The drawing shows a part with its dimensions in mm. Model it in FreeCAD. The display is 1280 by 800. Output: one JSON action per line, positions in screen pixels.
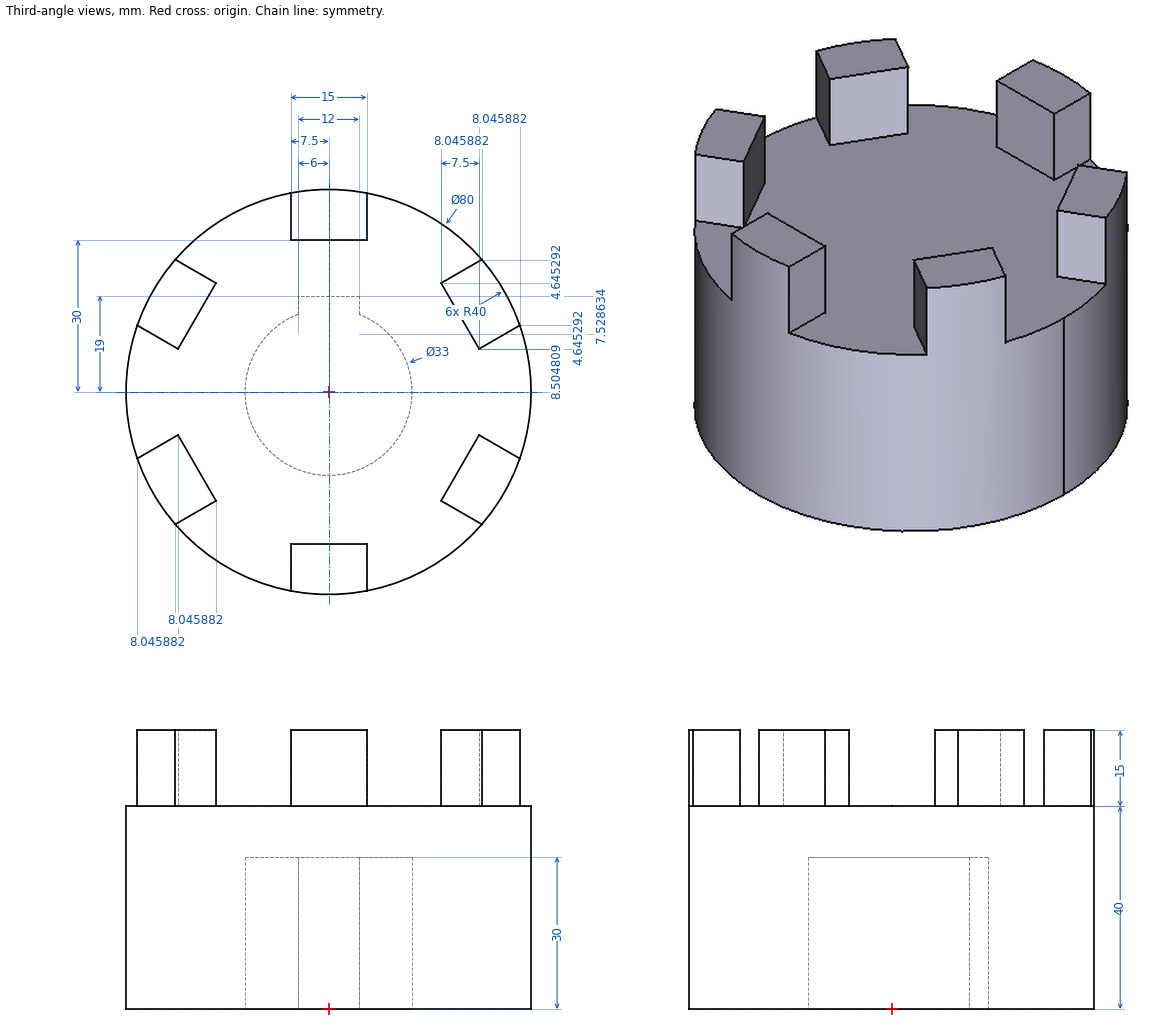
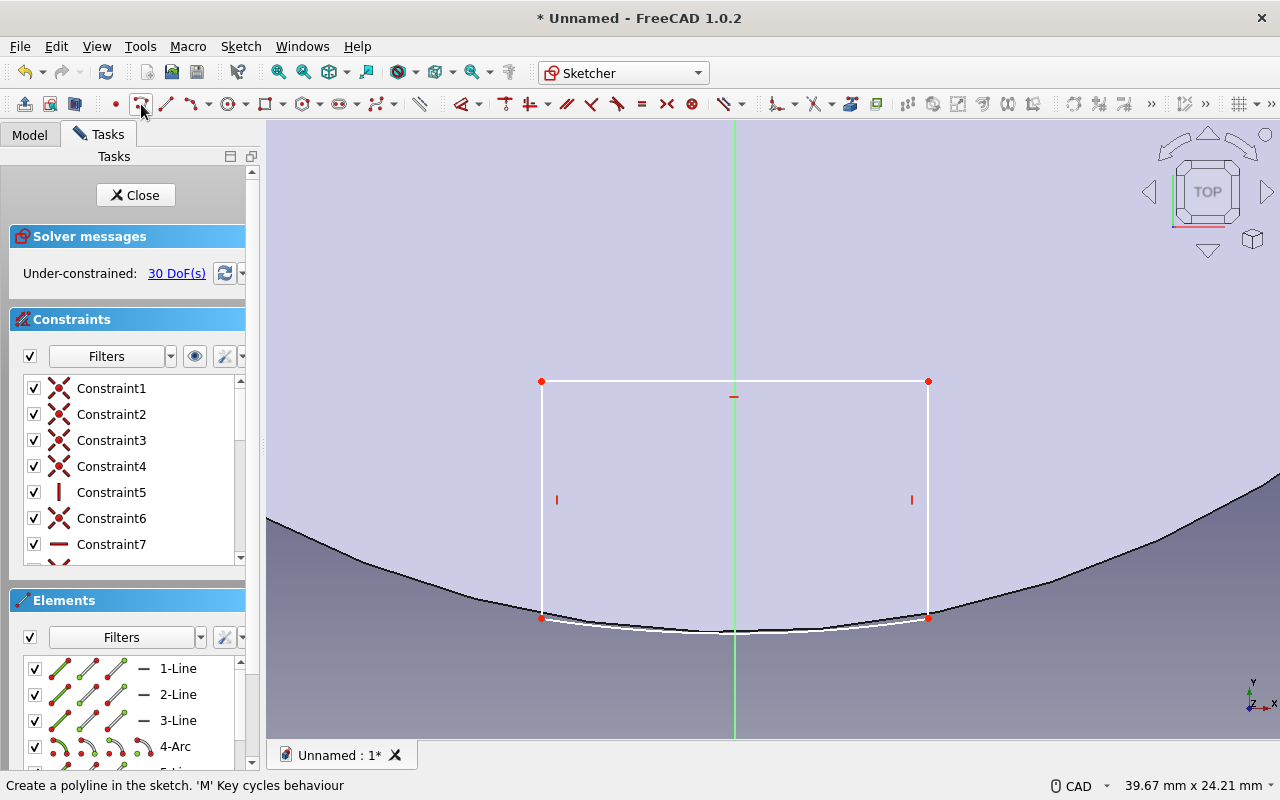
{"action": "scroll", "coordinate": [697, 637], "scroll_direction": "down", "scroll_amount": 8}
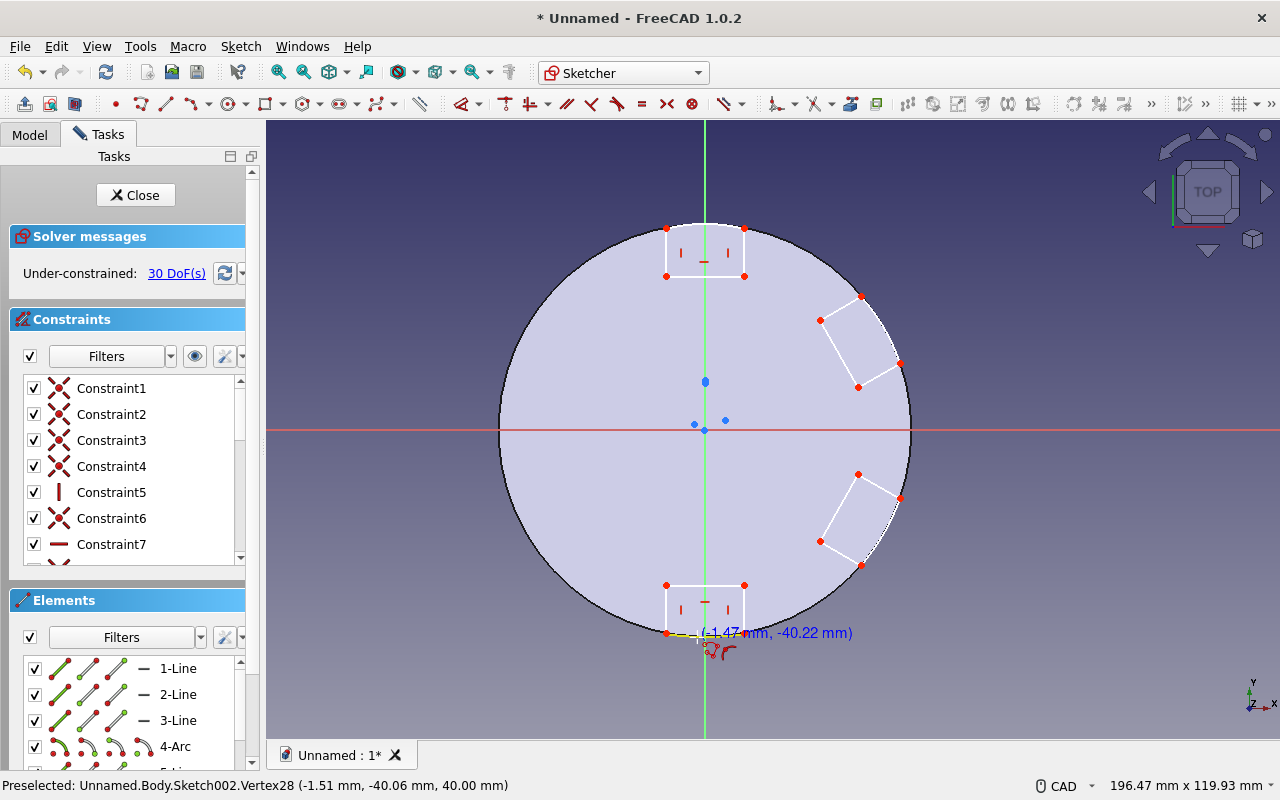
{"action": "left_click", "coordinate": [549, 565]}
{"action": "left_click", "coordinate": [590, 541]}
{"action": "left_click", "coordinate": [551, 474]}
{"action": "left_click", "coordinate": [510, 498]}
{"action": "right_click", "coordinate": [510, 498]}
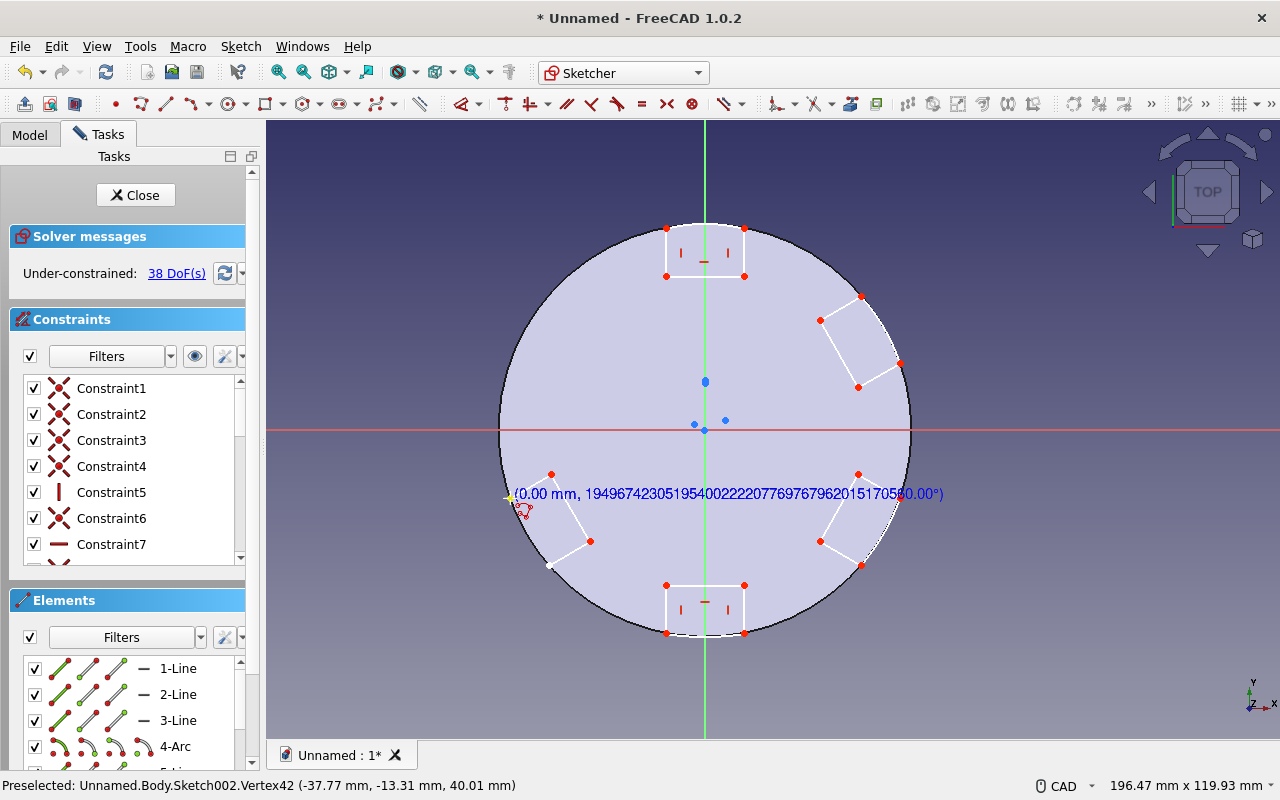
{"action": "key", "text": "g 3 a"}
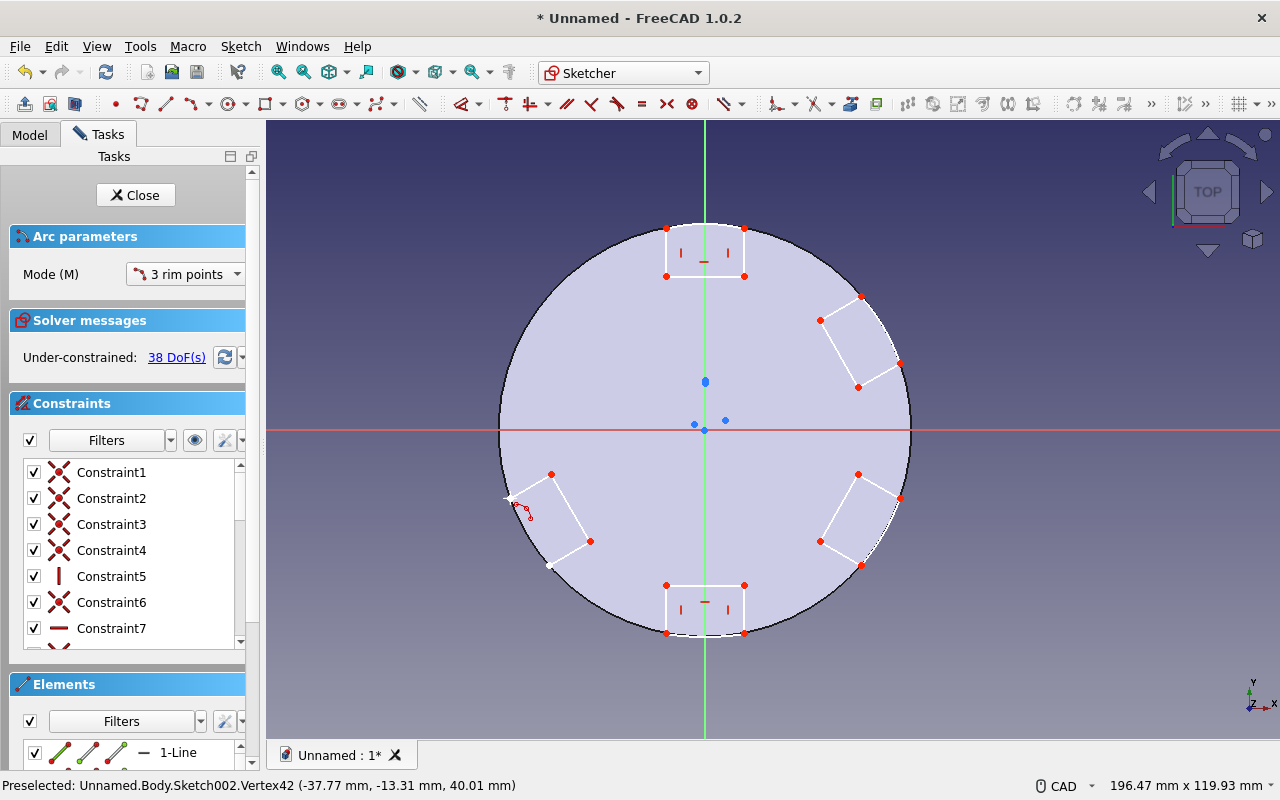
{"action": "left_click", "coordinate": [510, 499]}
{"action": "left_click", "coordinate": [549, 566]}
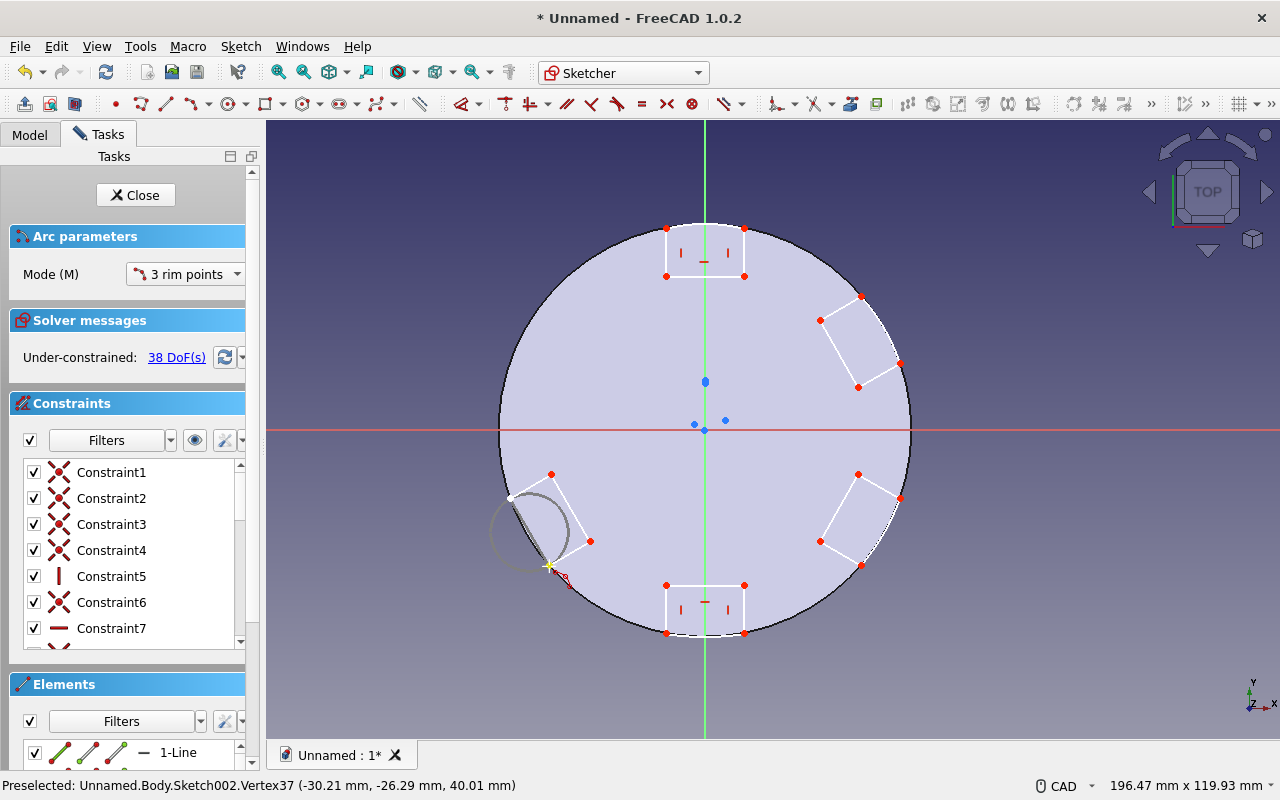
{"action": "scroll", "coordinate": [526, 534], "scroll_direction": "up", "scroll_amount": 8}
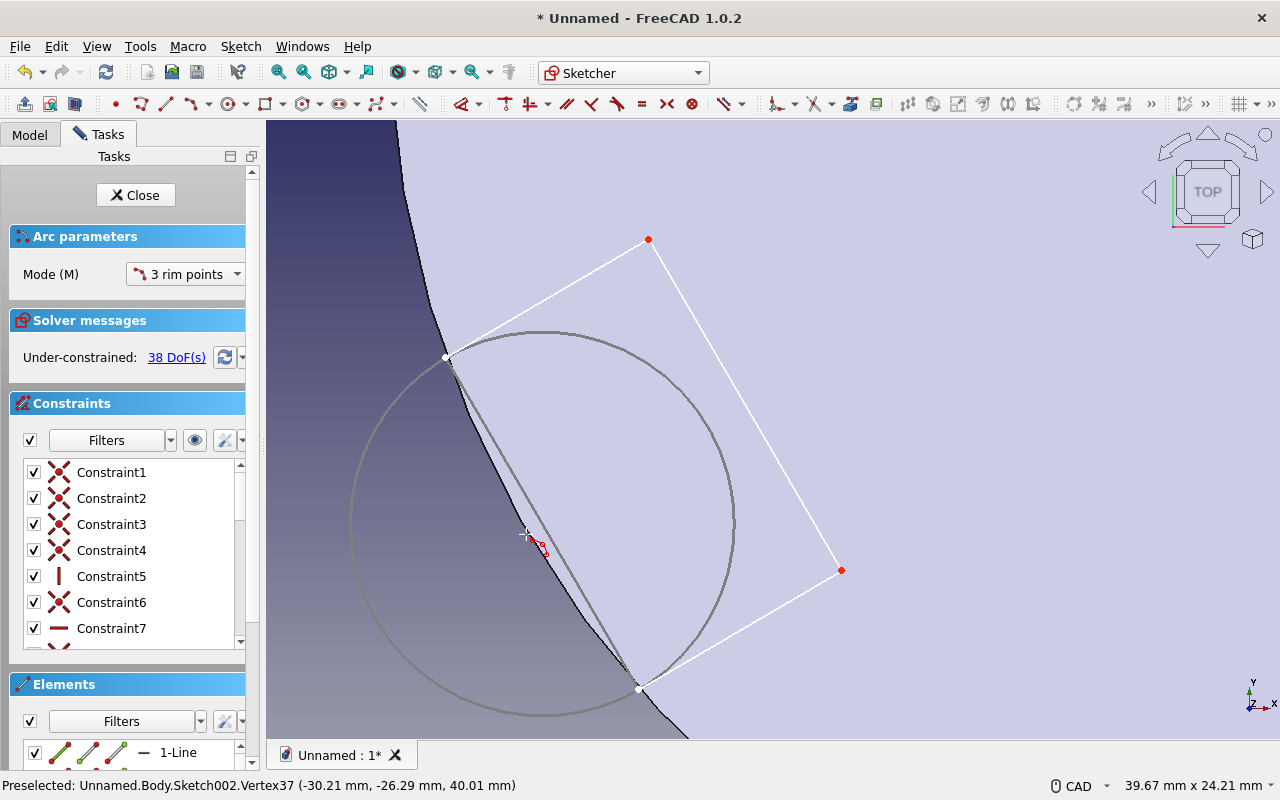
{"action": "left_click", "coordinate": [526, 529]}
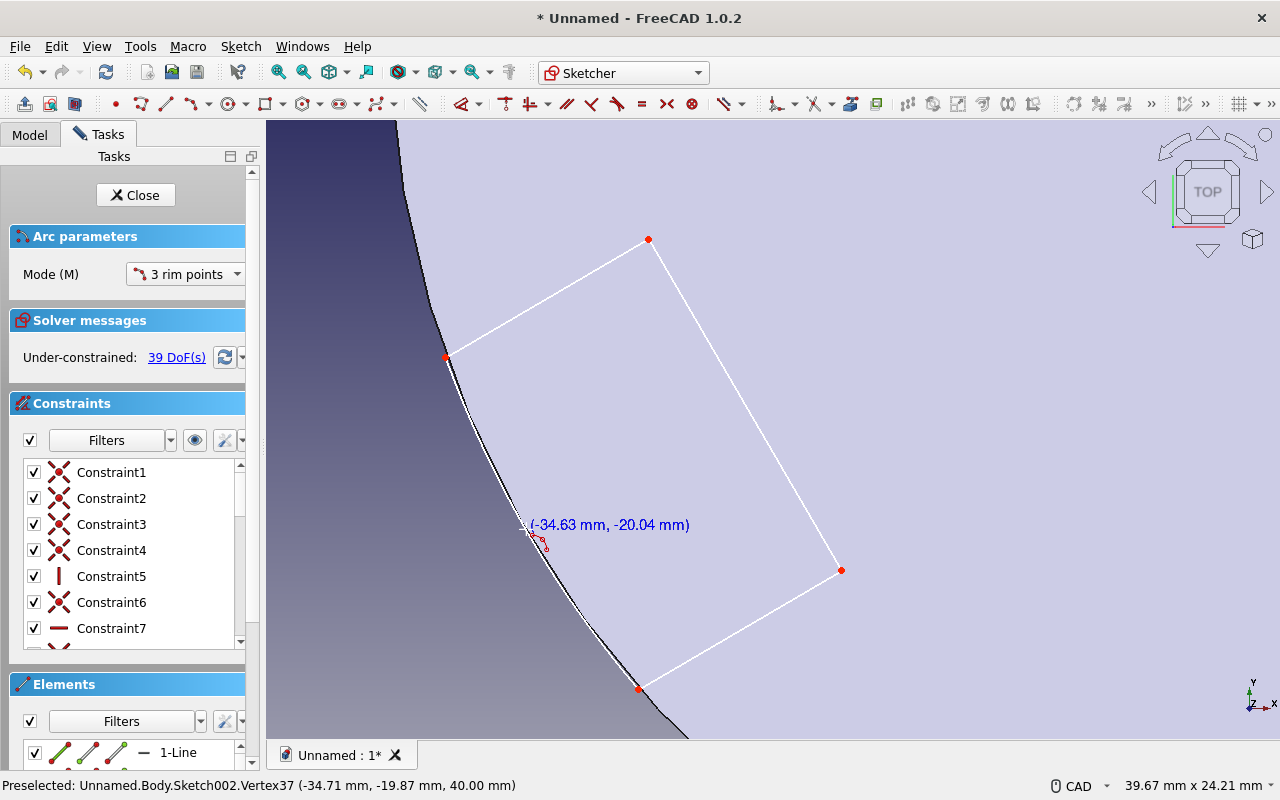
{"action": "key", "text": "g m"}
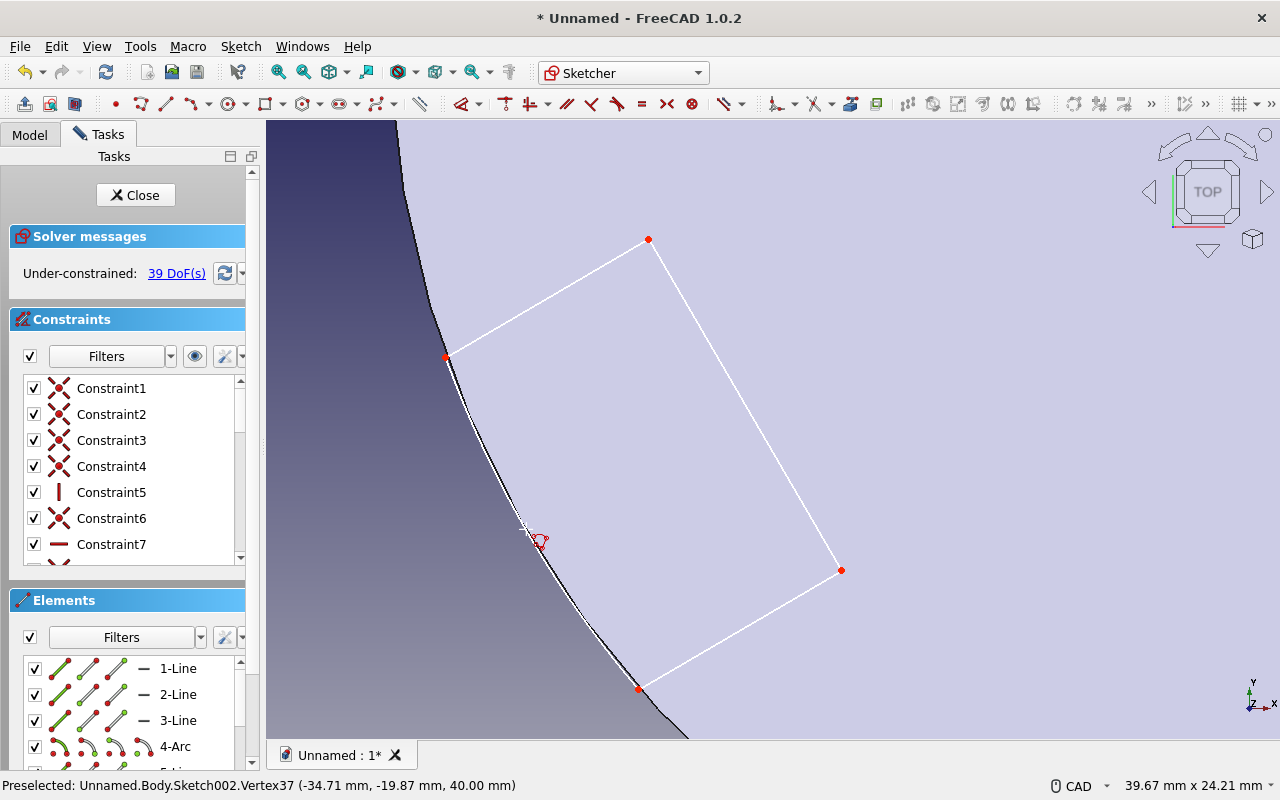
{"action": "scroll", "coordinate": [526, 534], "scroll_direction": "down", "scroll_amount": 8}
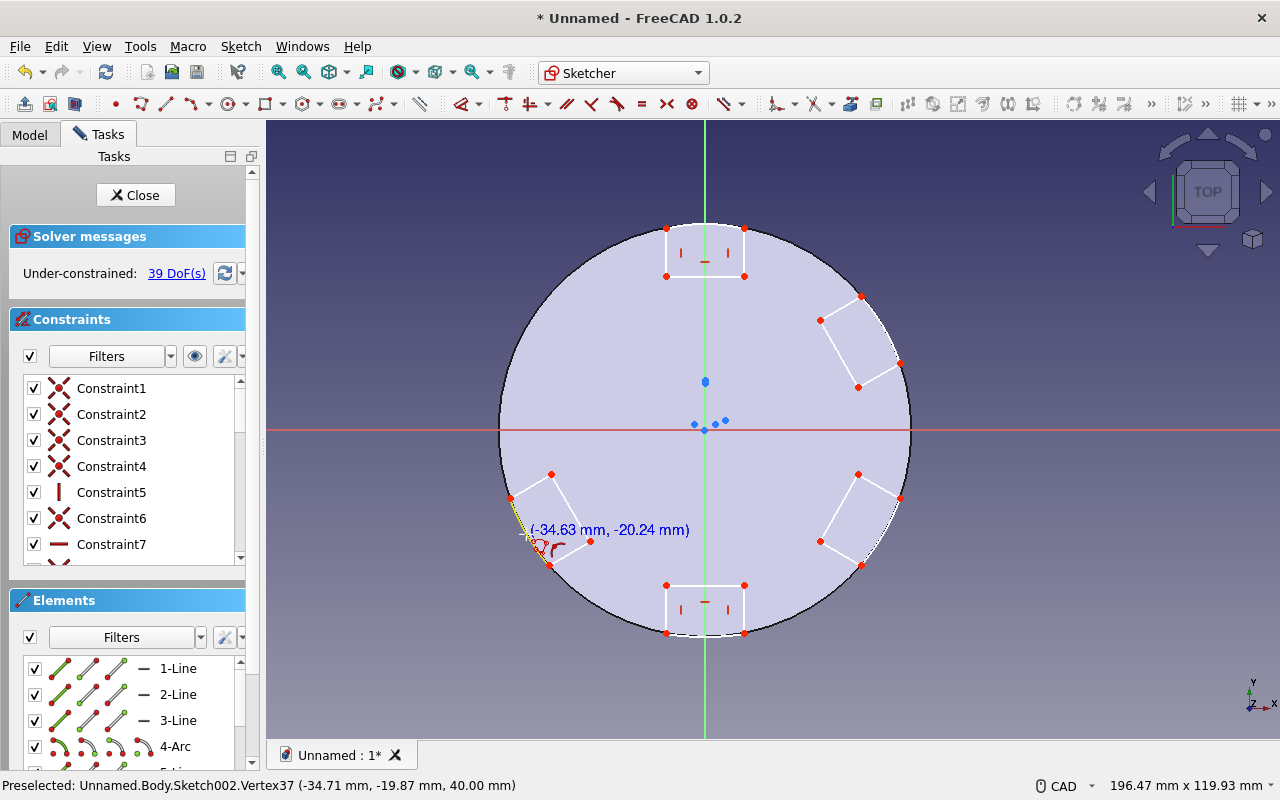
{"action": "left_click", "coordinate": [510, 362]}
{"action": "left_click", "coordinate": [551, 386]}
{"action": "left_click", "coordinate": [590, 319]}
{"action": "left_click", "coordinate": [549, 295]}
{"action": "right_click", "coordinate": [549, 295]}